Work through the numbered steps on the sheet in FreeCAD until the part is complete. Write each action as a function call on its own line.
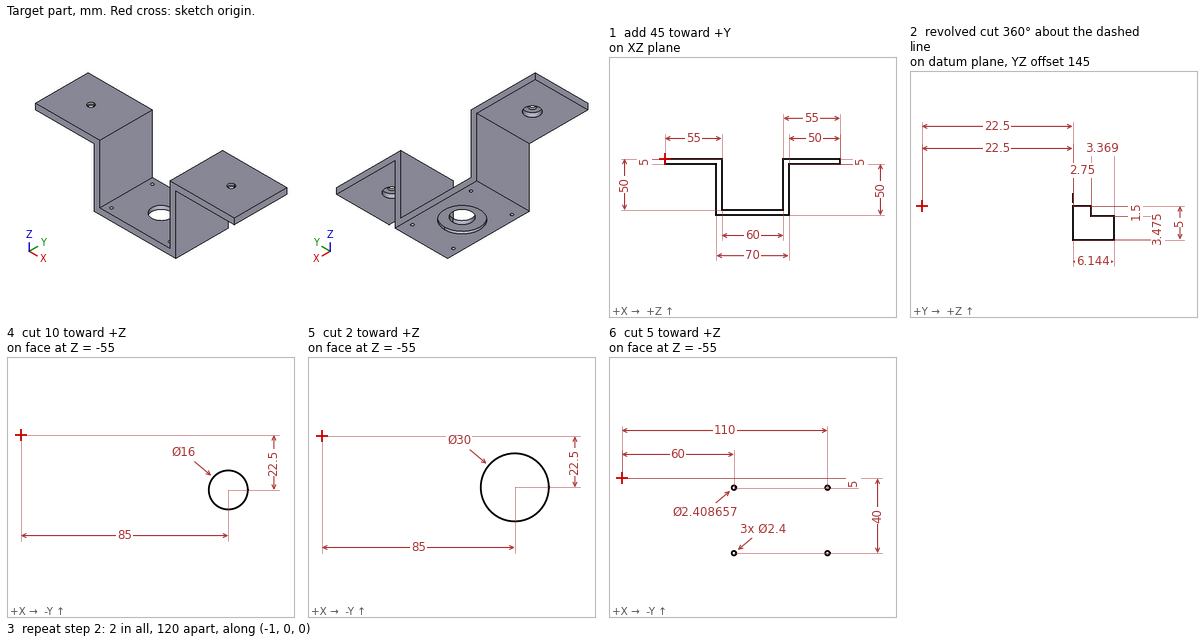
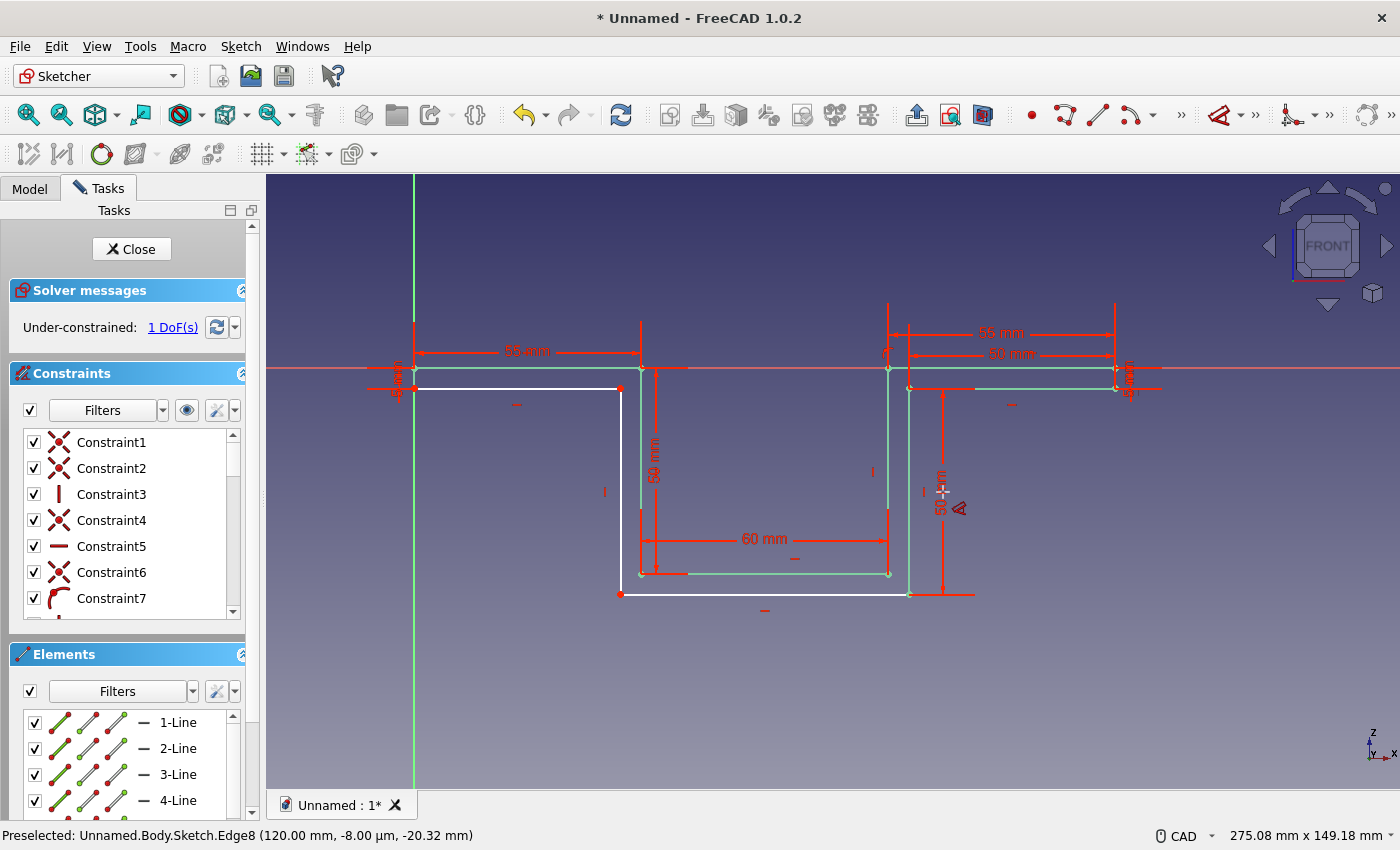
click(823, 595)
click(765, 629)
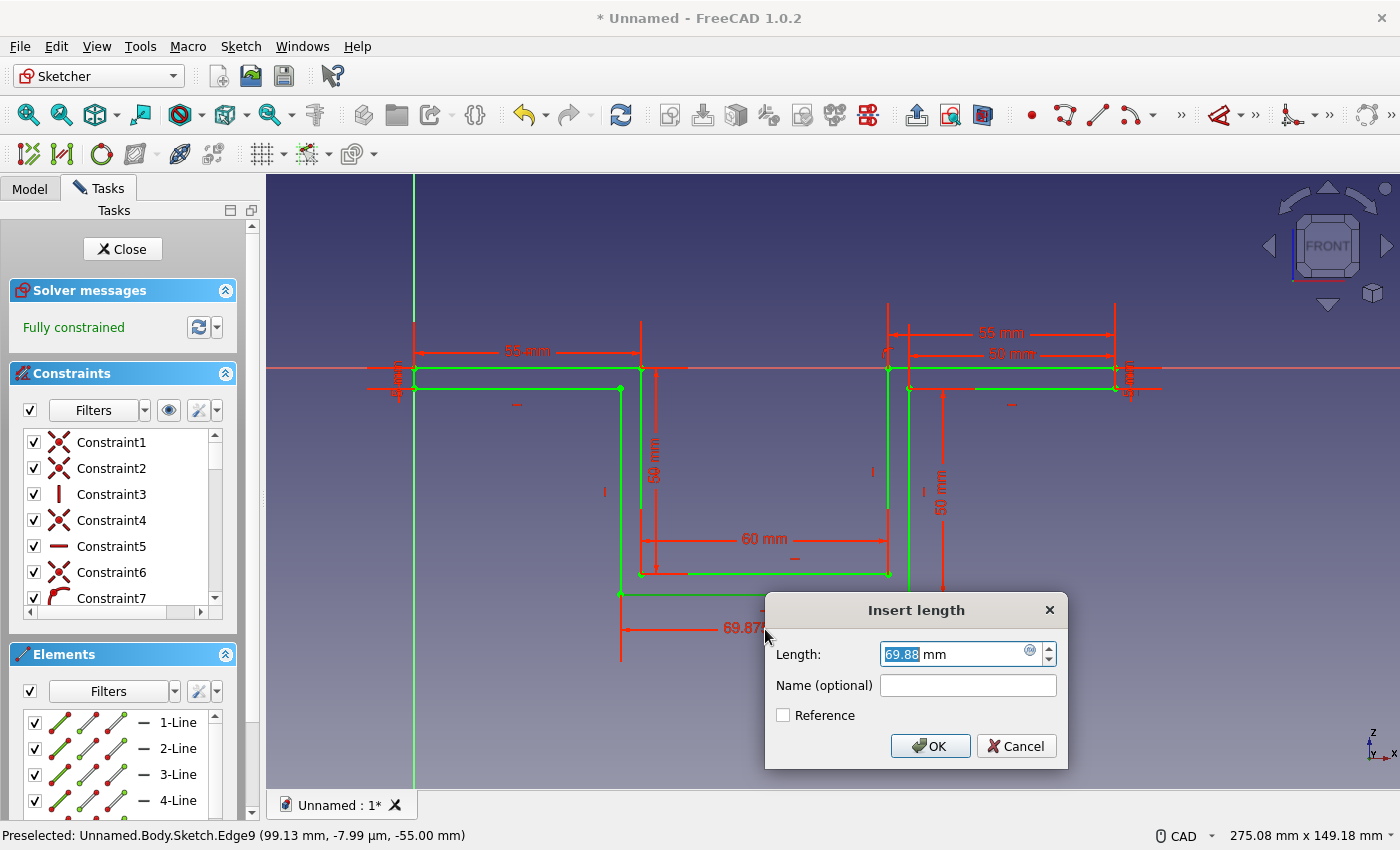
text(70)
key(Return)
key(Escape)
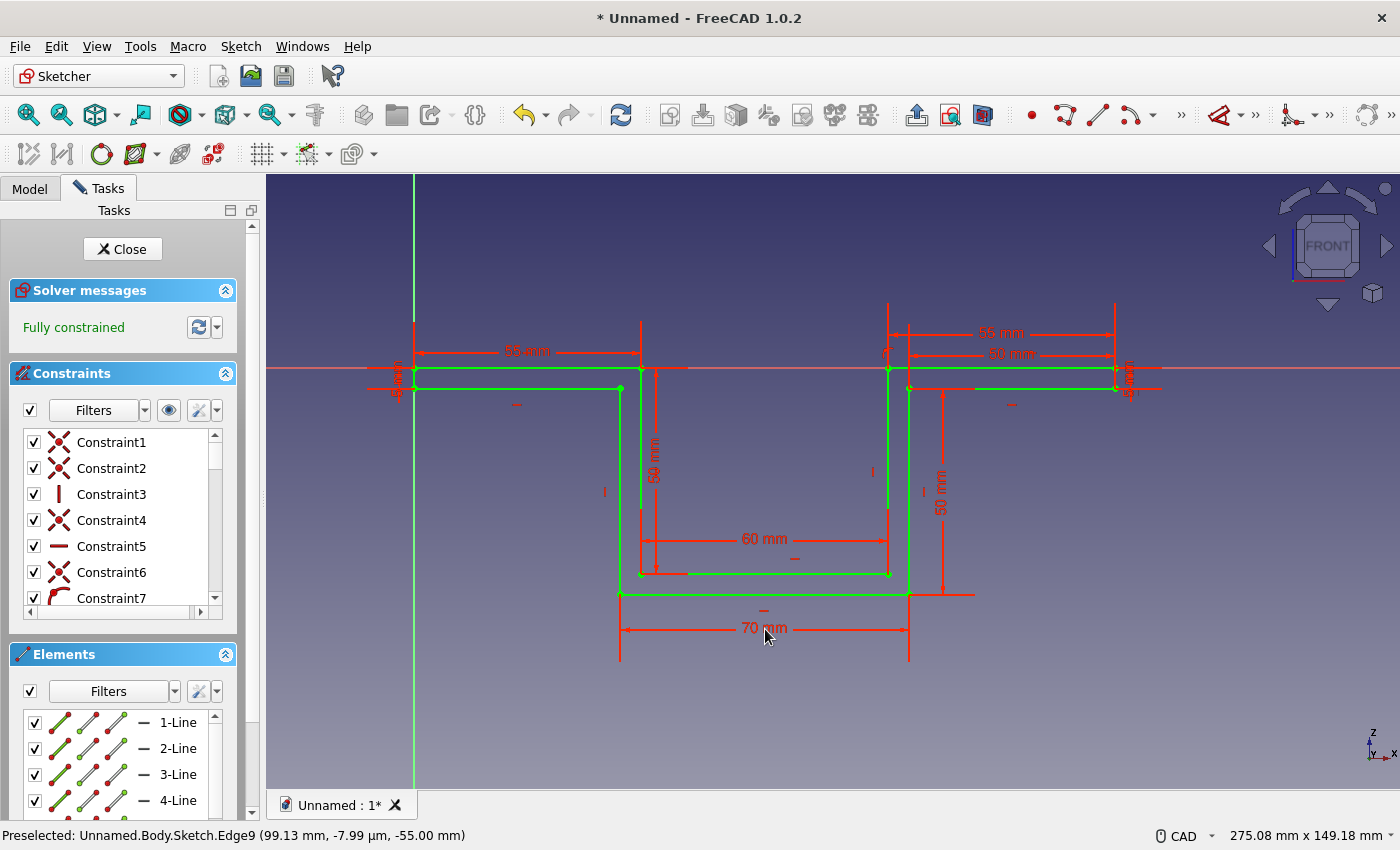
click(123, 249)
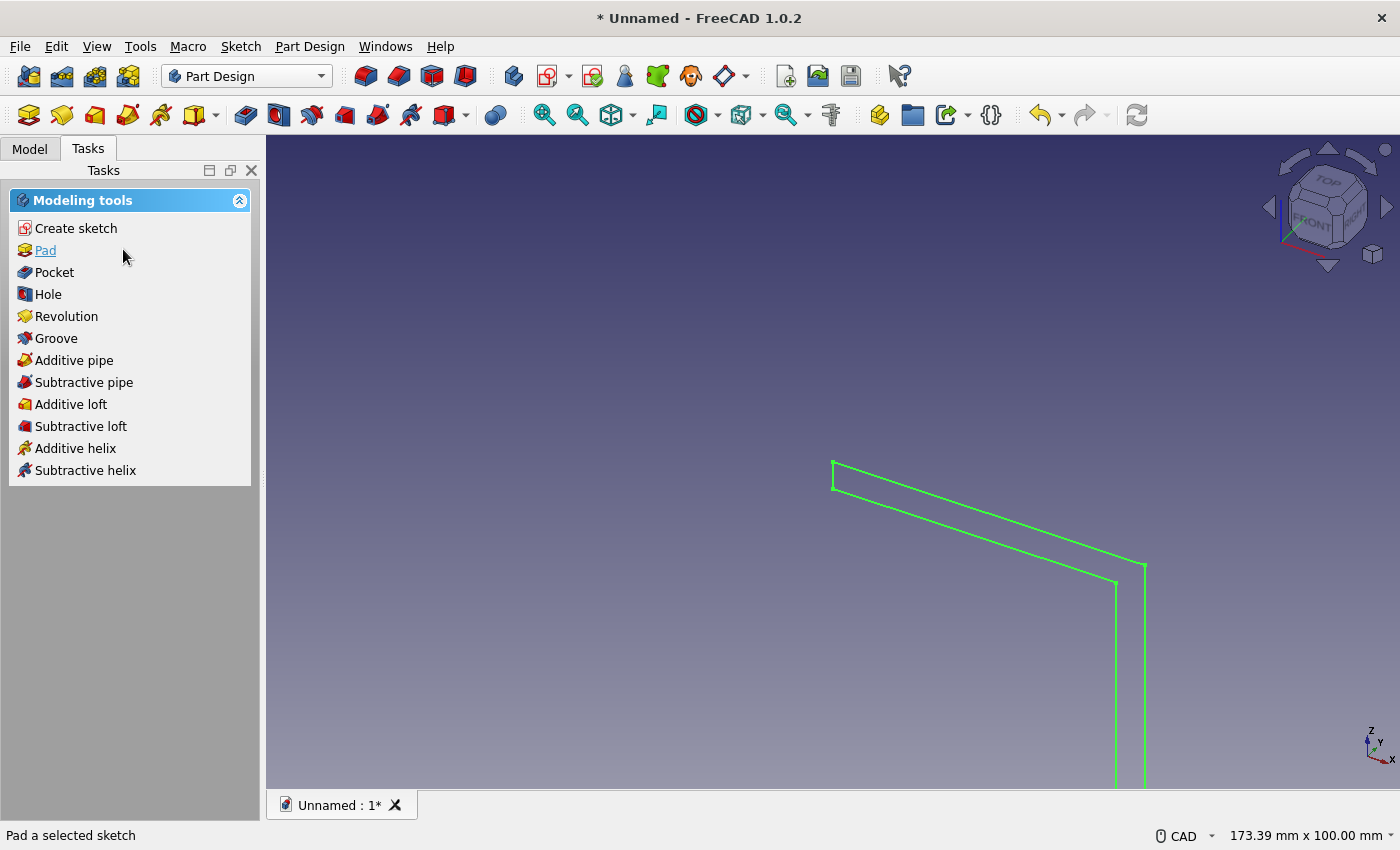
click(29, 116)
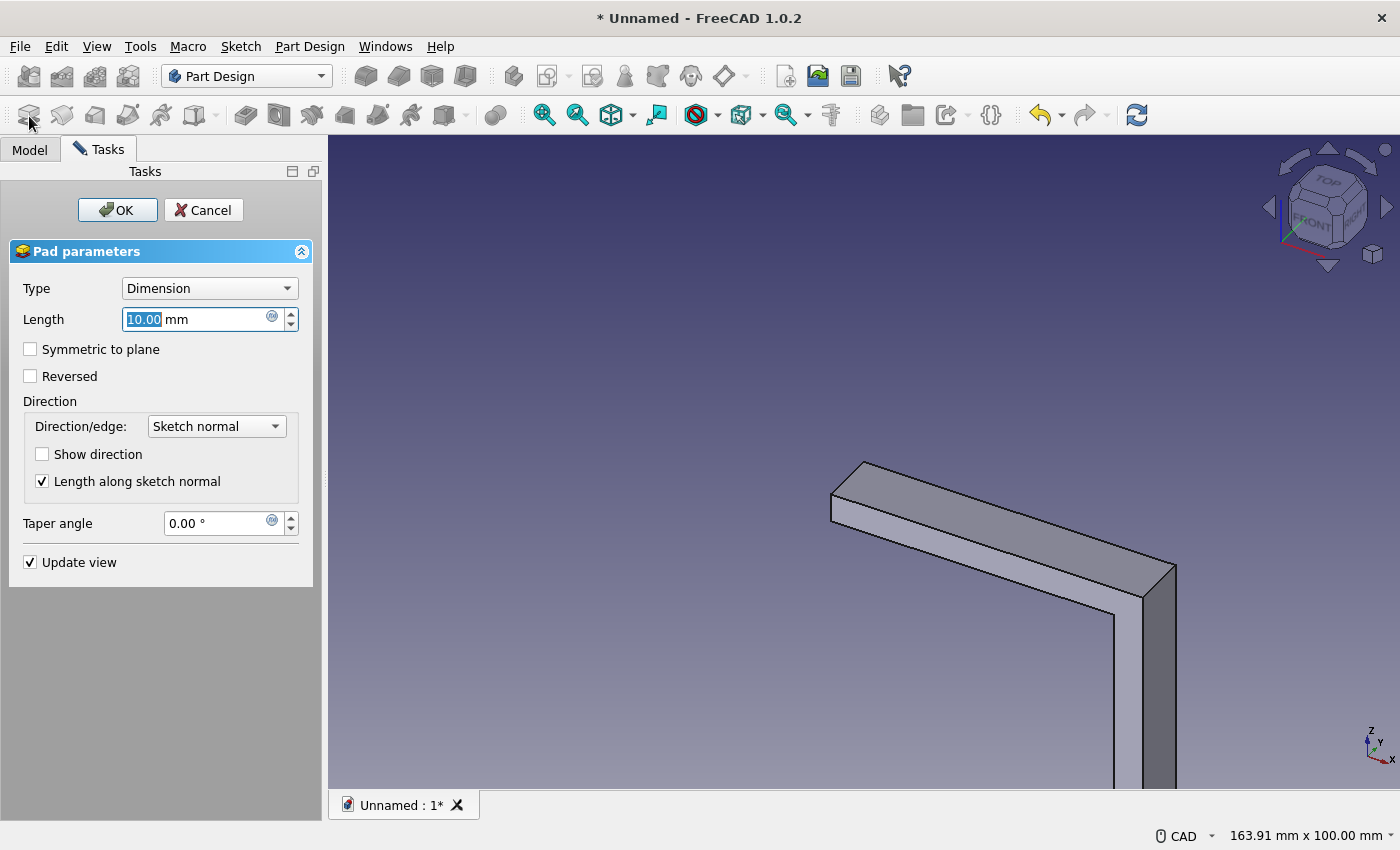
text(45)
key(Tab)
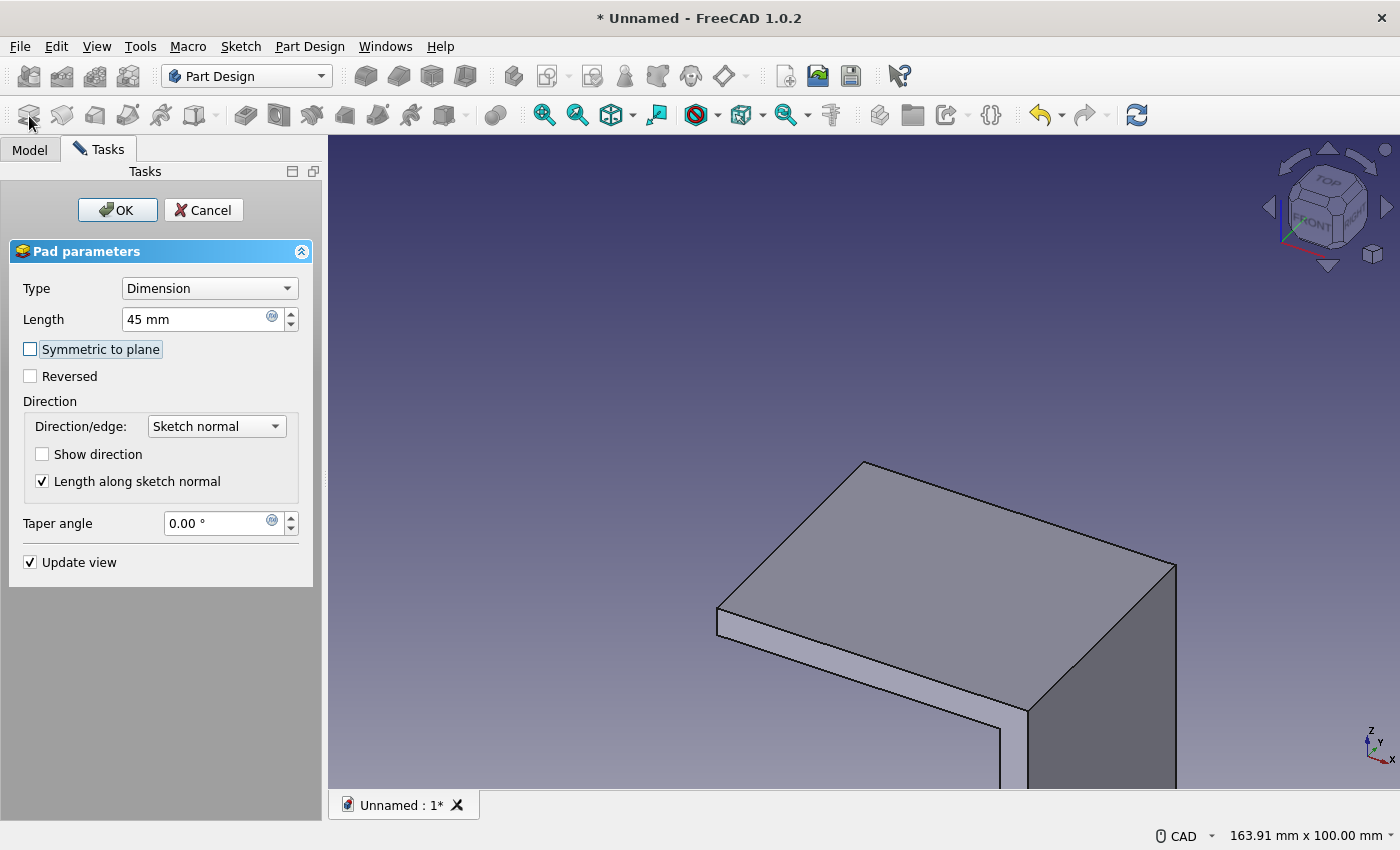
click(31, 376)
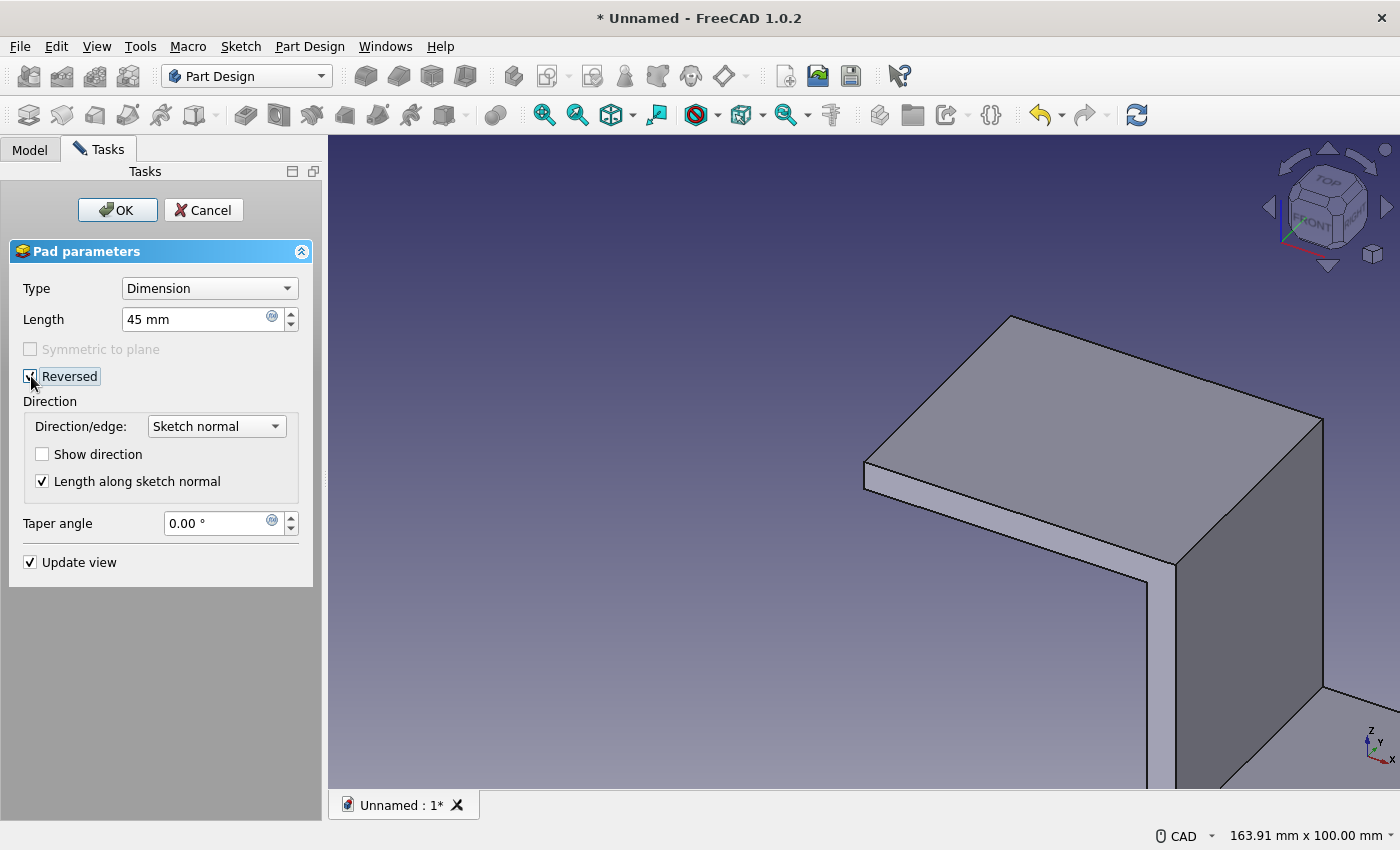
click(118, 210)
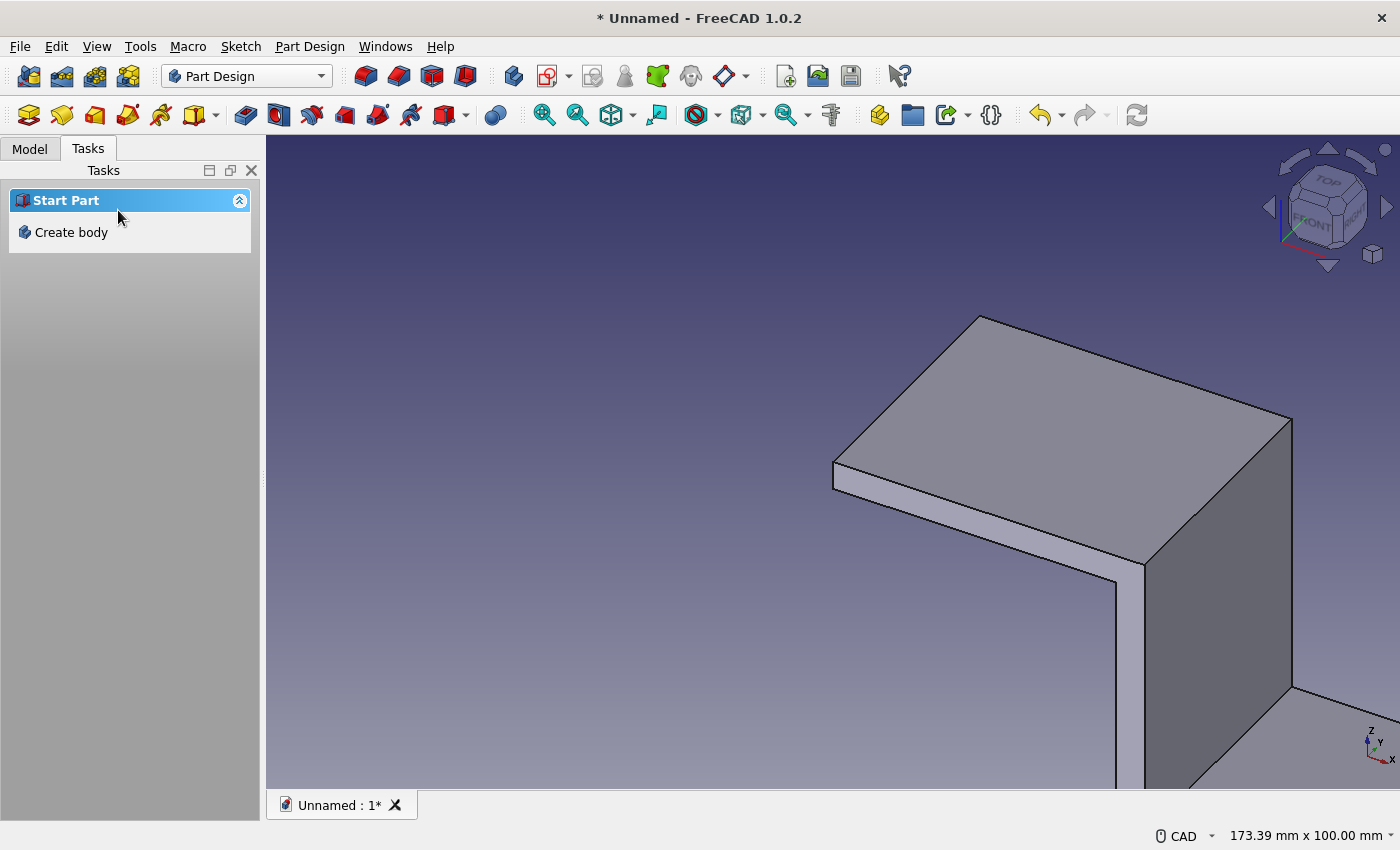
click(545, 116)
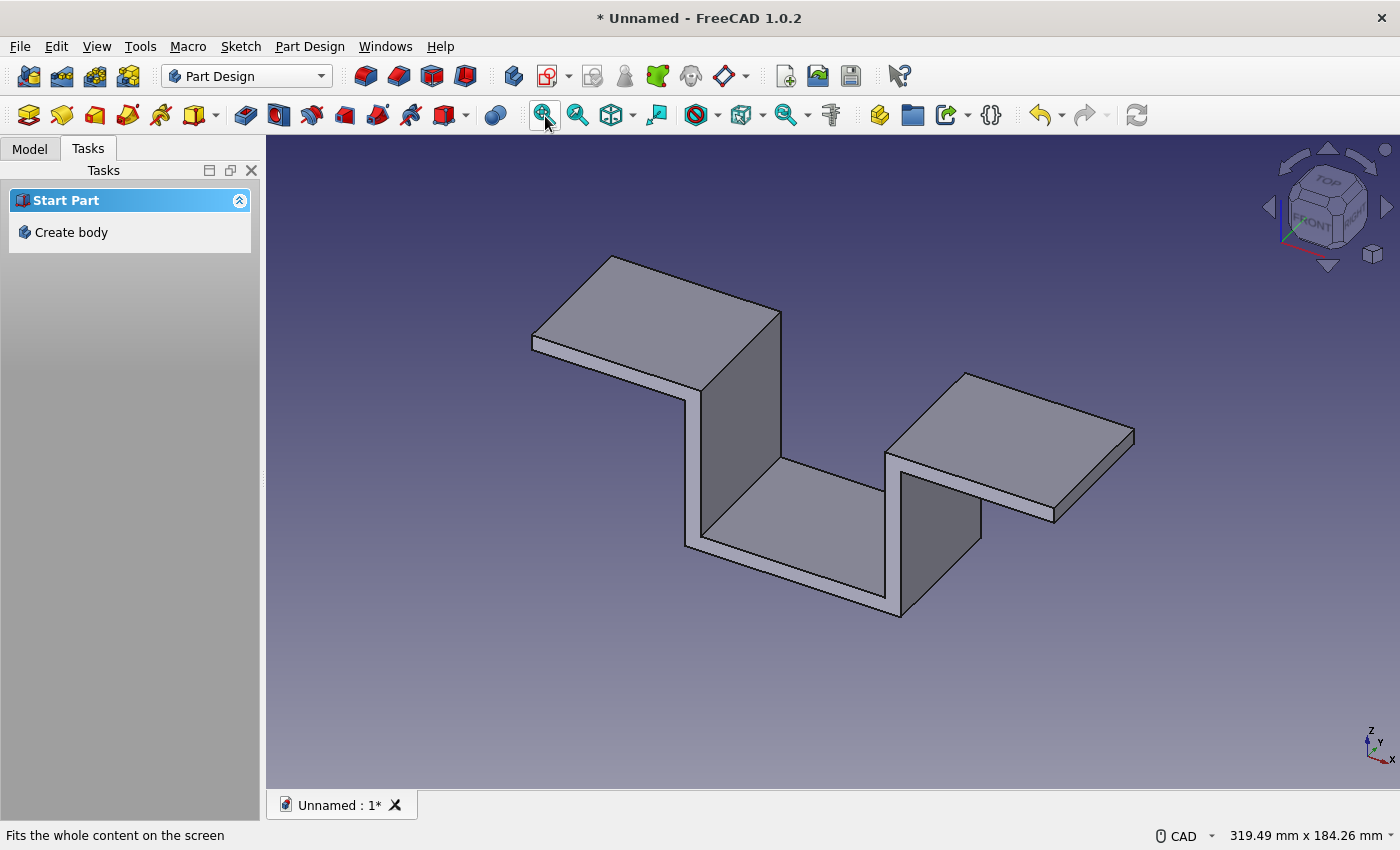
click(30, 148)